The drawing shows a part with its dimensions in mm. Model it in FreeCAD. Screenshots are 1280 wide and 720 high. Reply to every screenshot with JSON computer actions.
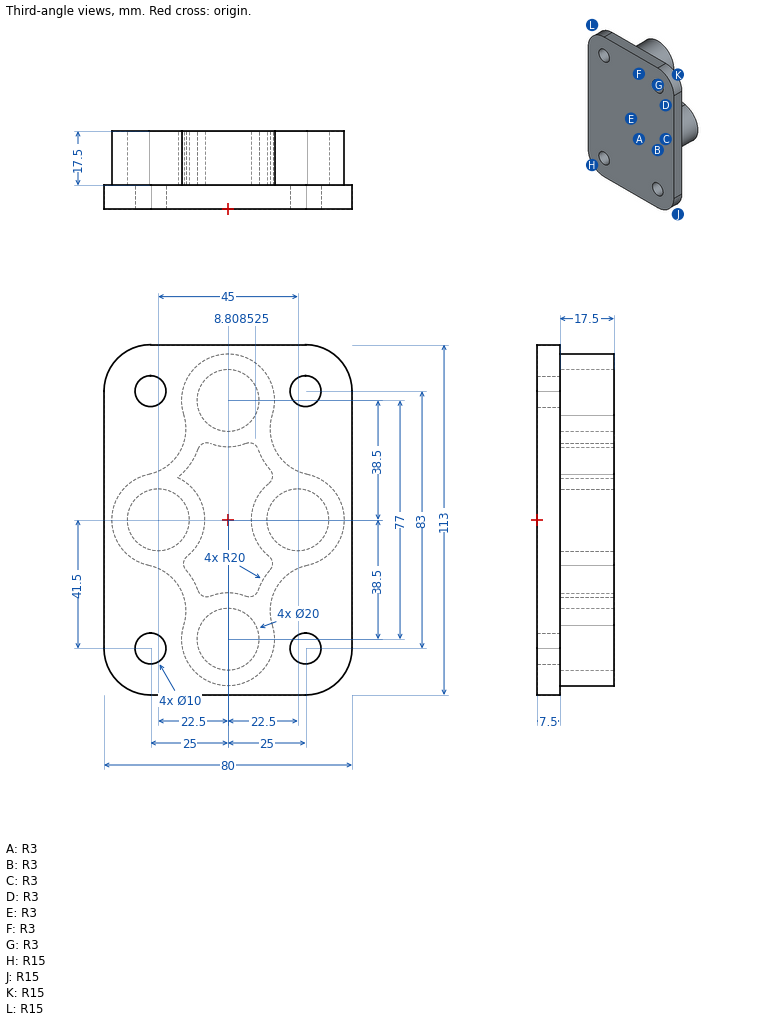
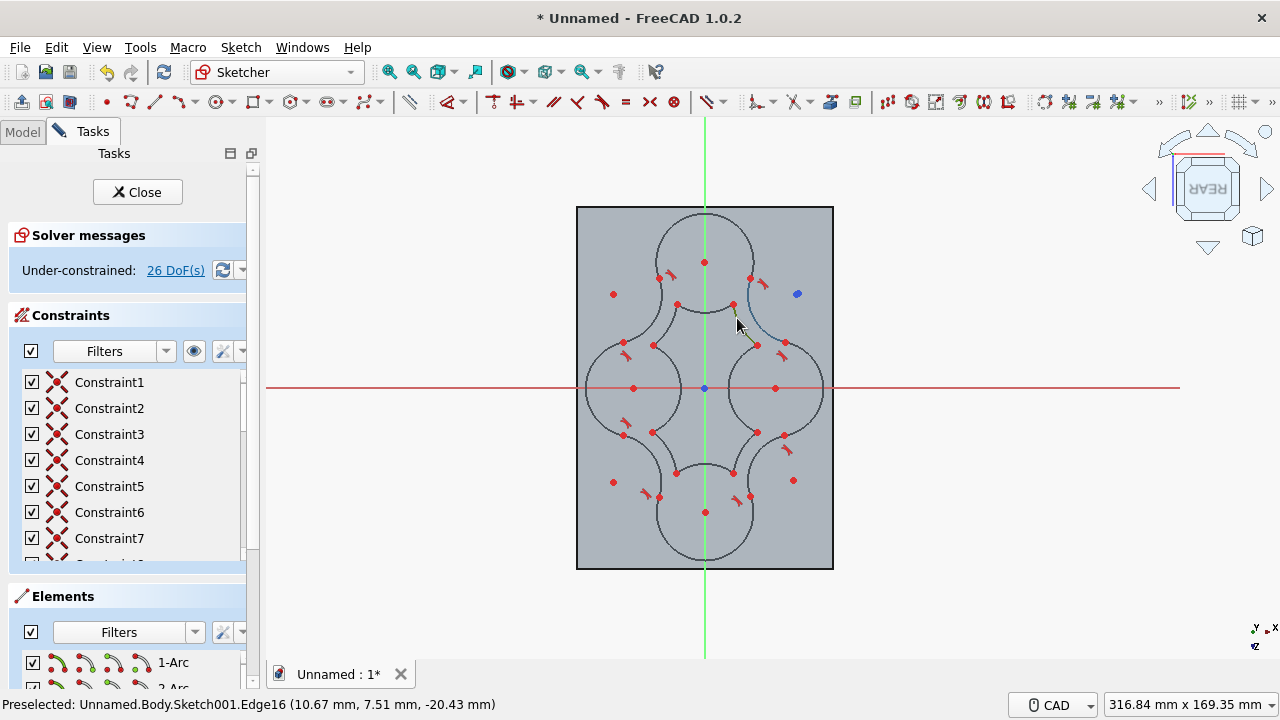
{"action": "key", "text": "c"}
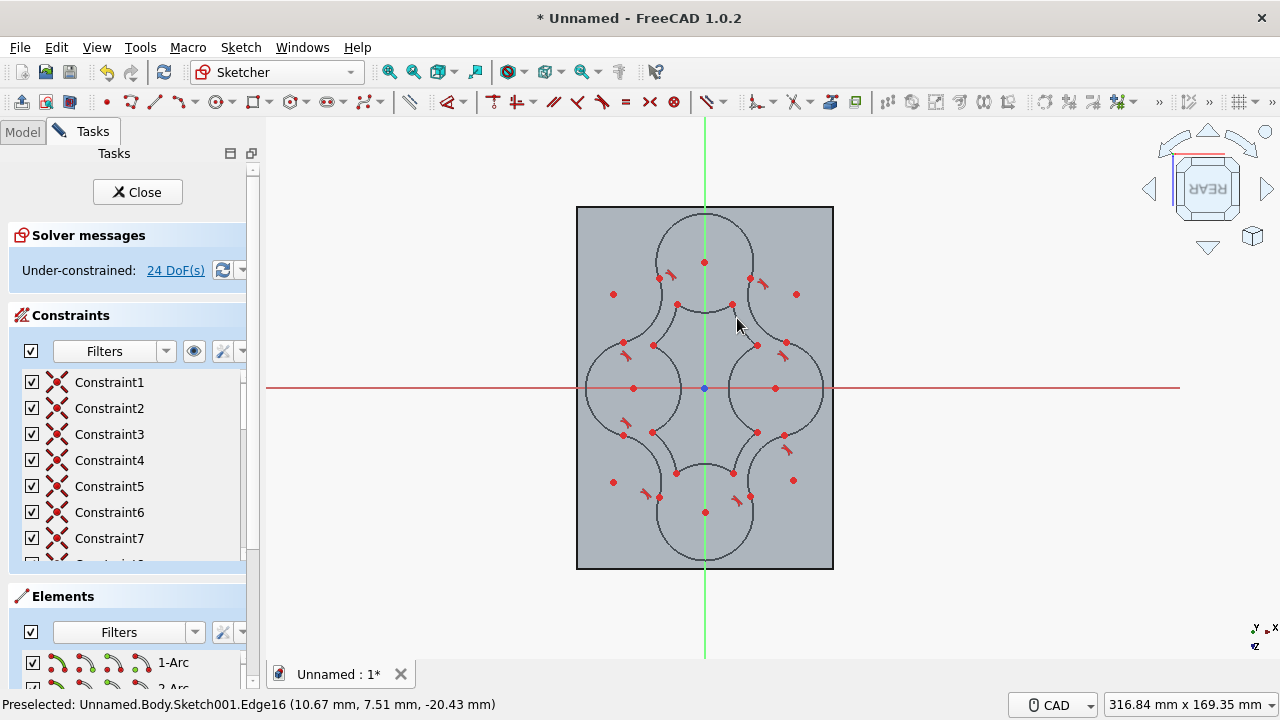
{"action": "left_click", "coordinate": [593, 364]}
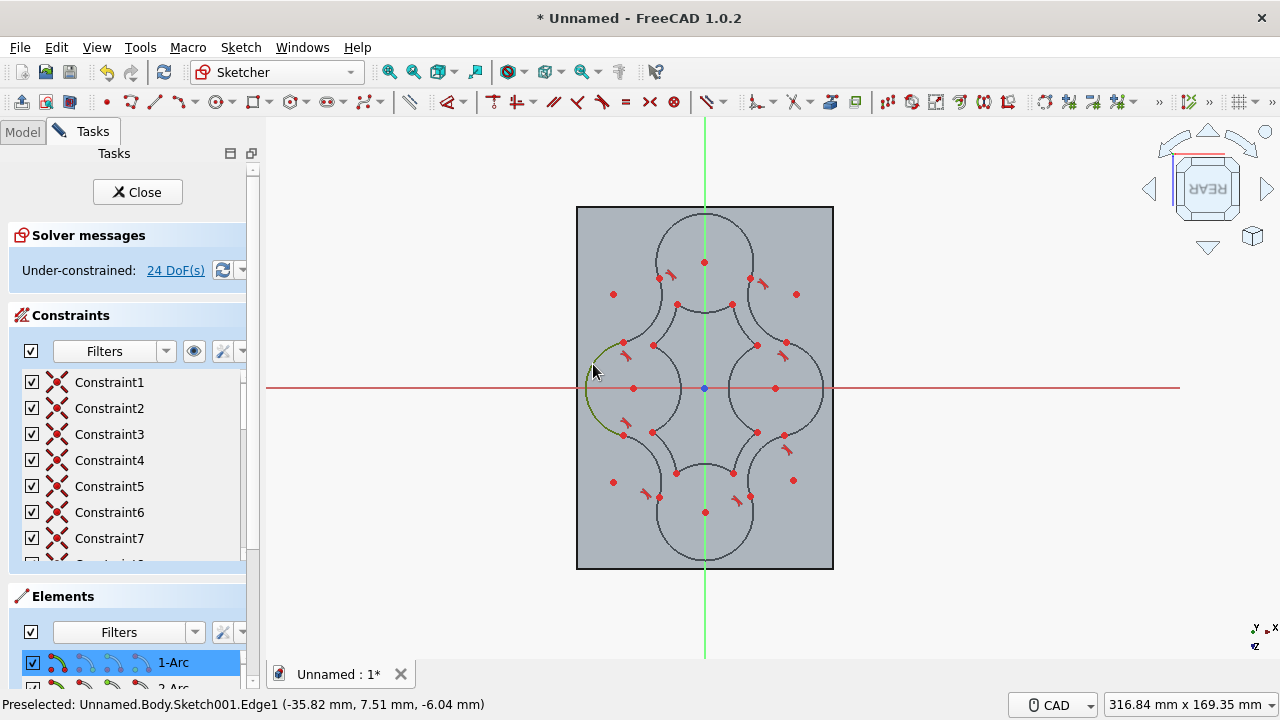
{"action": "left_click", "coordinate": [661, 474]}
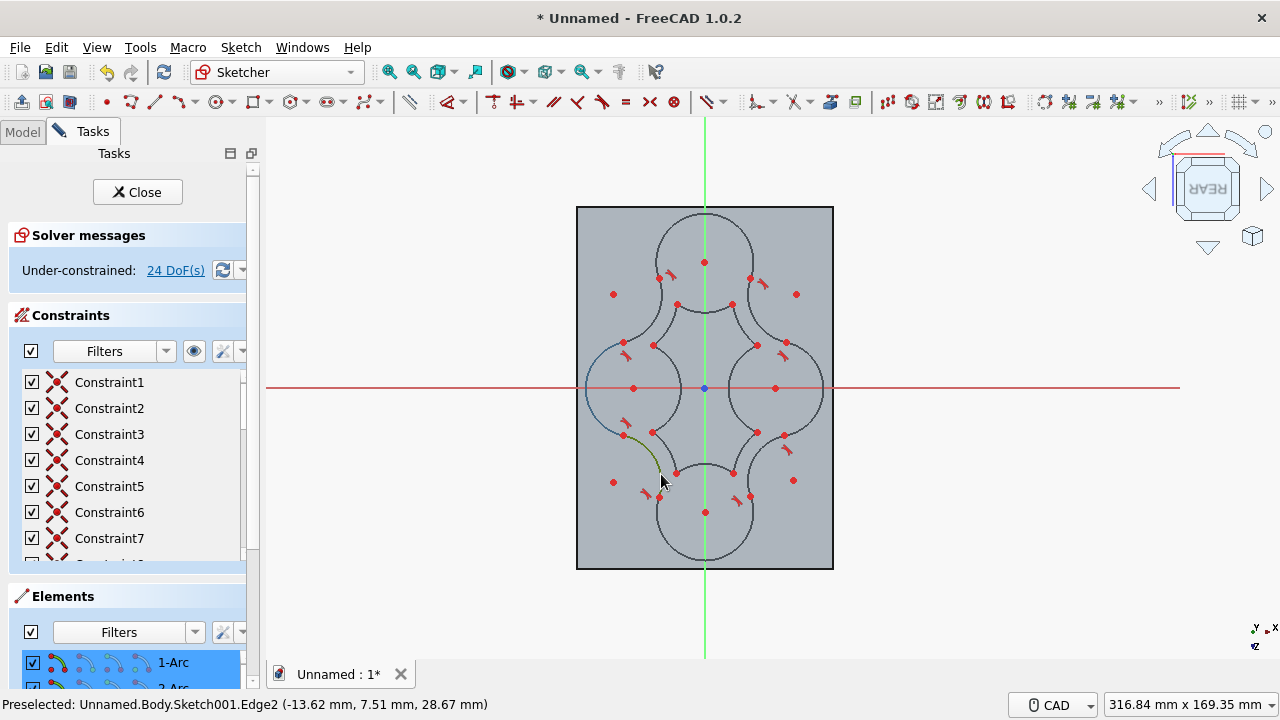
{"action": "left_click", "coordinate": [672, 548]}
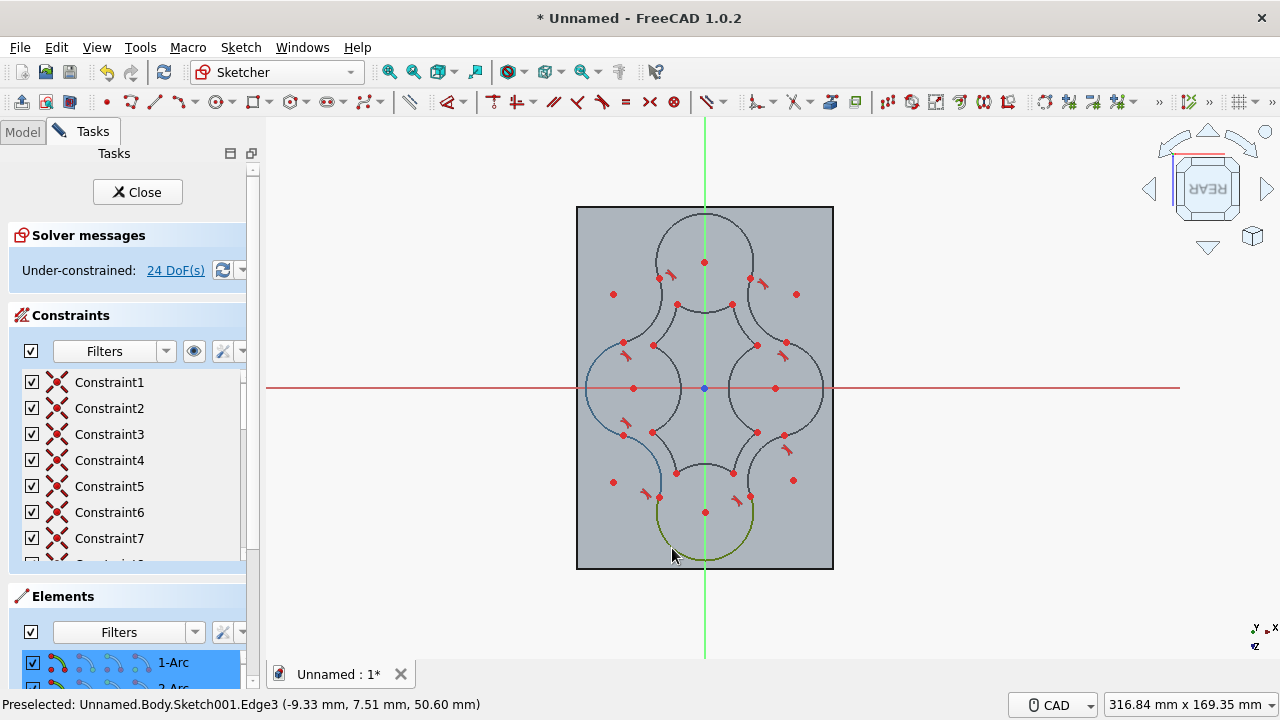
{"action": "left_click", "coordinate": [764, 446]}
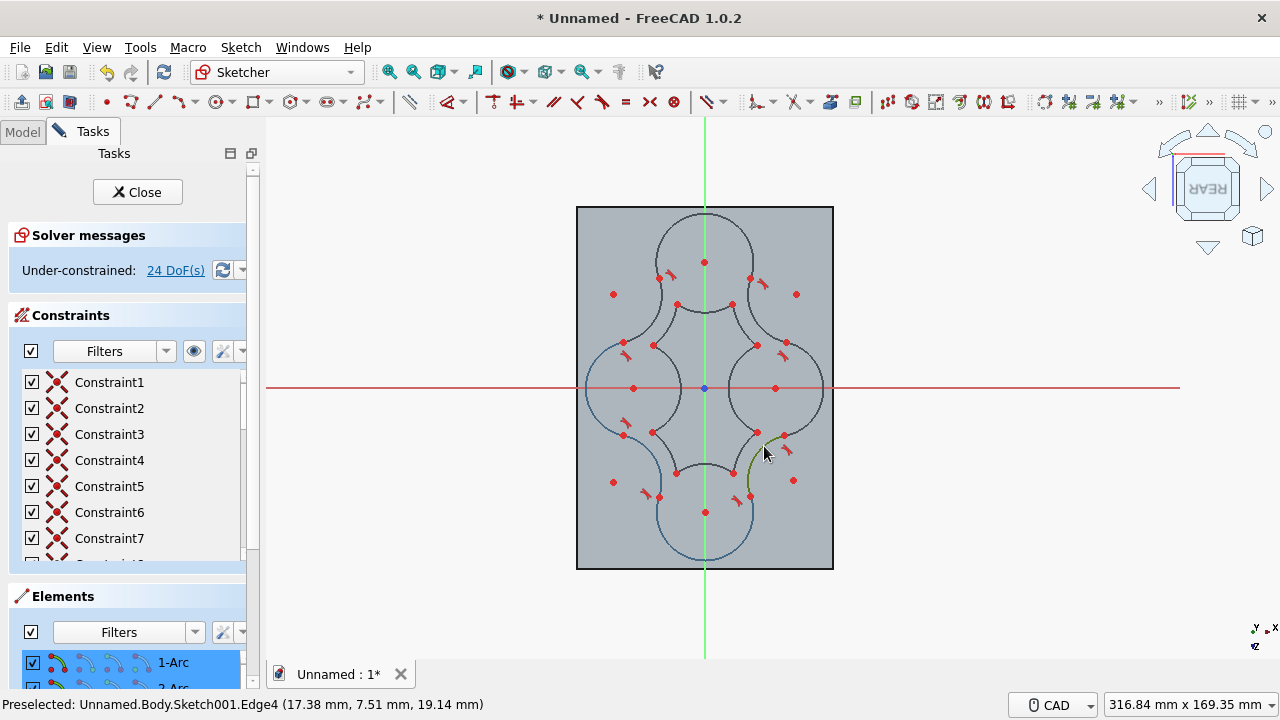
{"action": "left_click", "coordinate": [816, 414]}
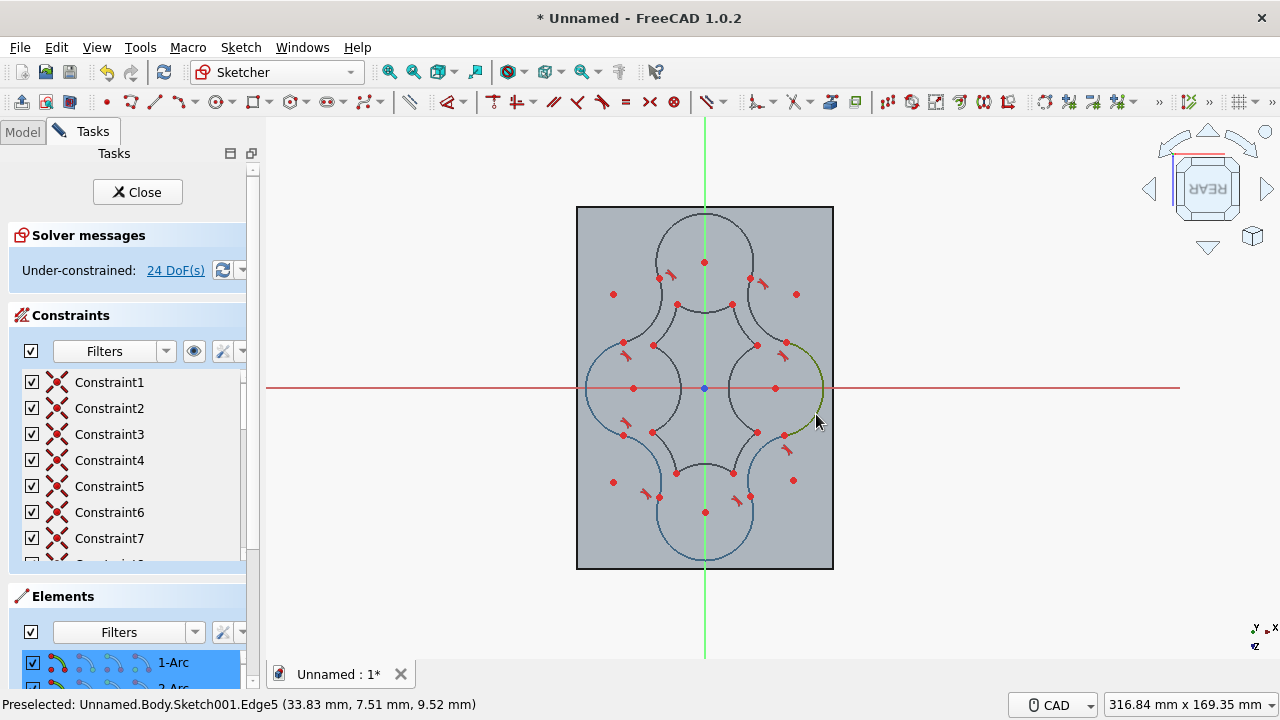
{"action": "left_click", "coordinate": [749, 303]}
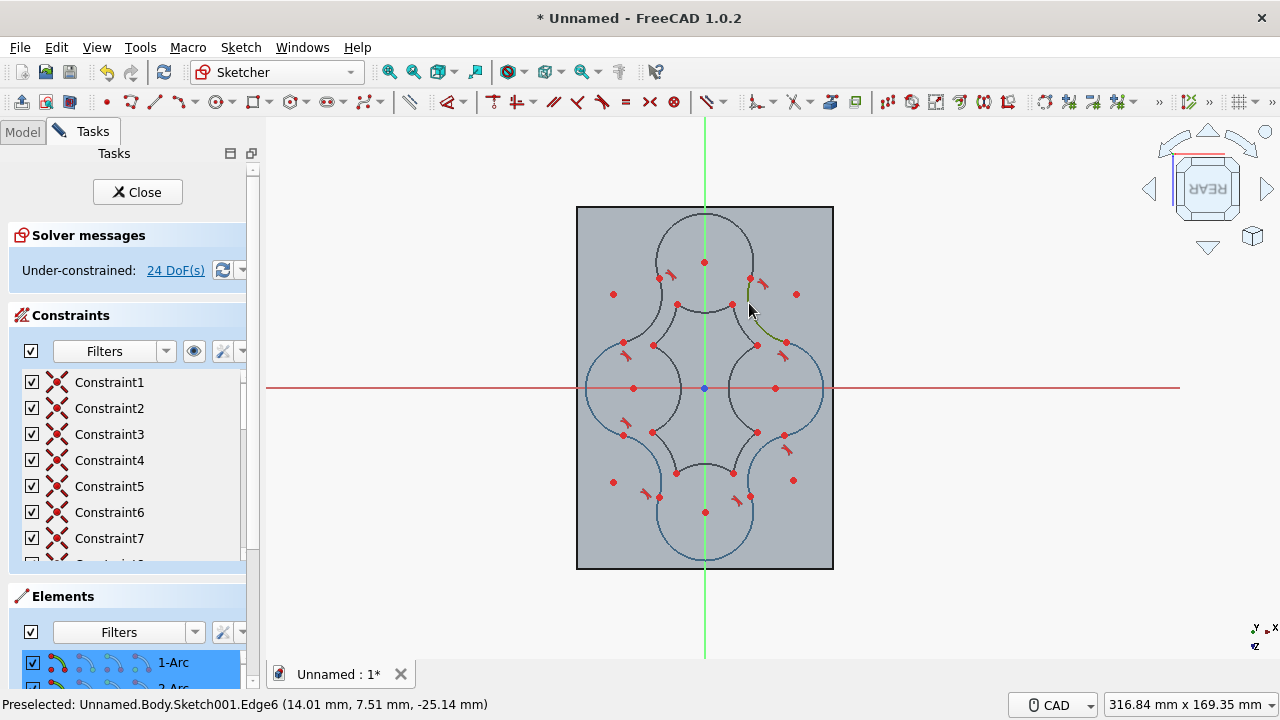
{"action": "left_click", "coordinate": [738, 227]}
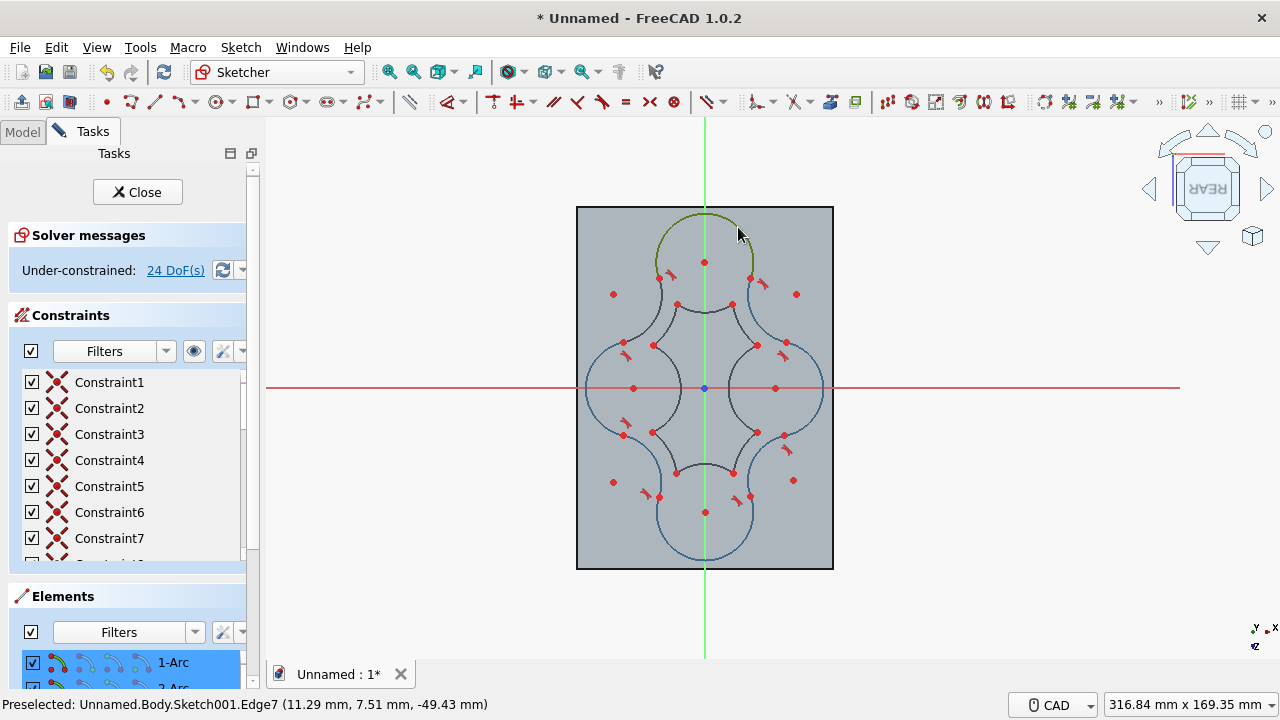
{"action": "left_click", "coordinate": [645, 331]}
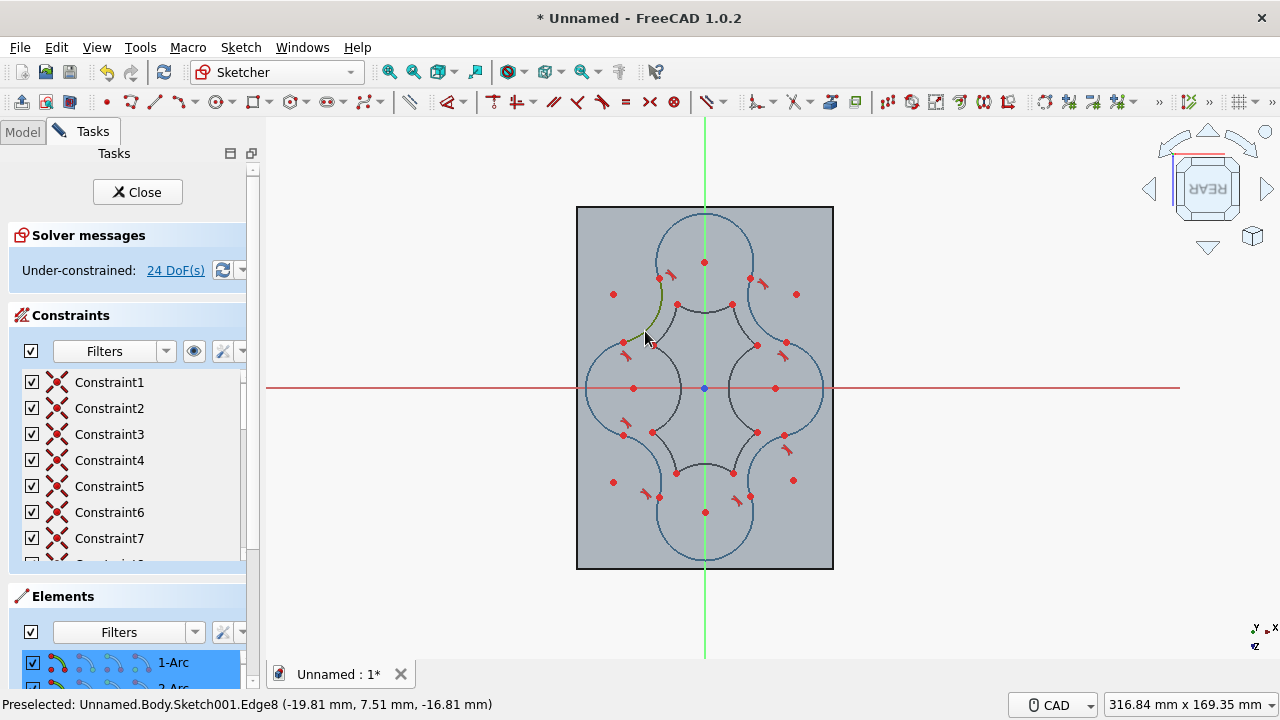
{"action": "left_click", "coordinate": [734, 368]}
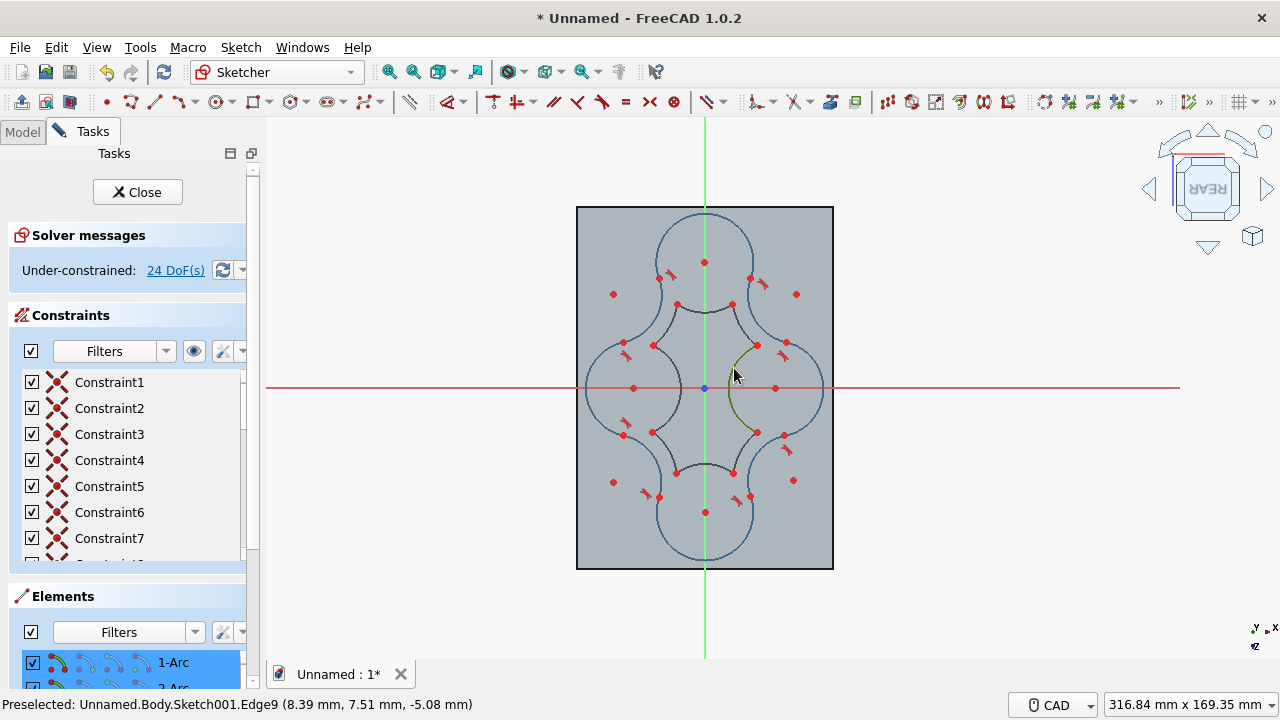
{"action": "left_click", "coordinate": [717, 466]}